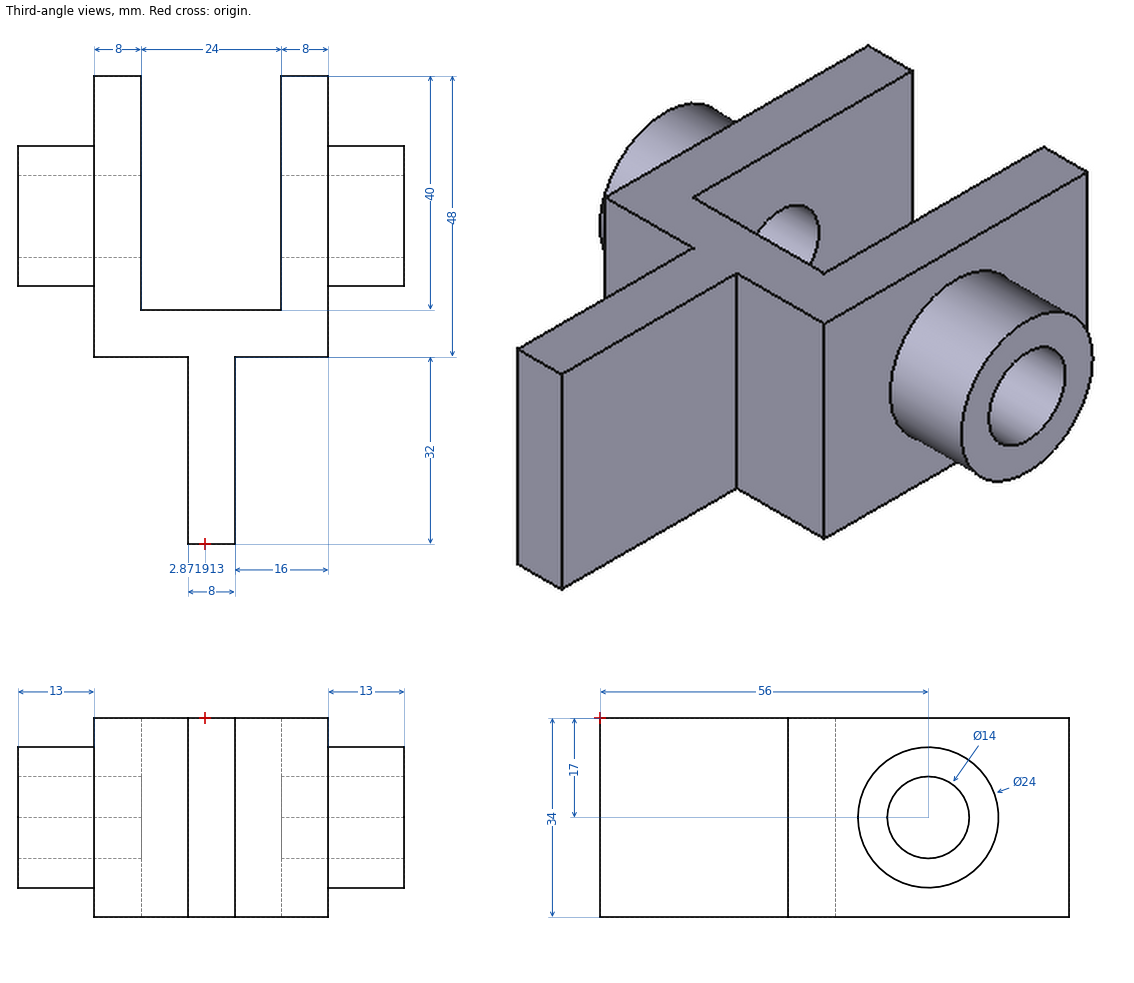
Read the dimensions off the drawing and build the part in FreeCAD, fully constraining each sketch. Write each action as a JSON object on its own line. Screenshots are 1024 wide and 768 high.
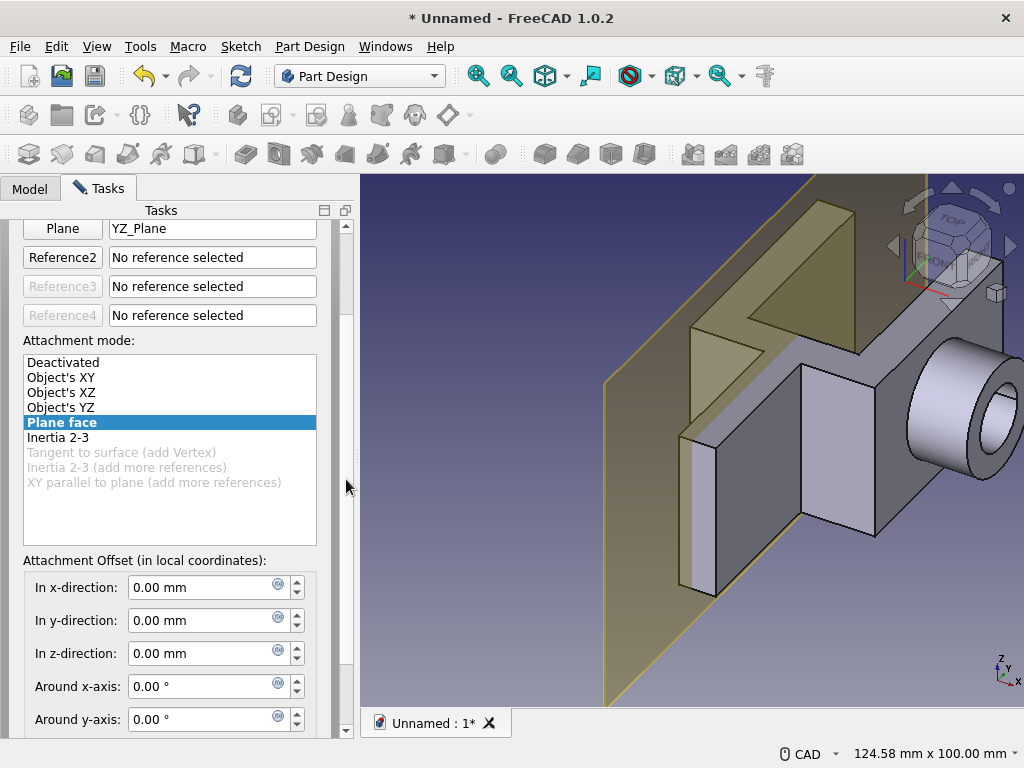
{"action": "triple_click", "coordinate": [210, 654]}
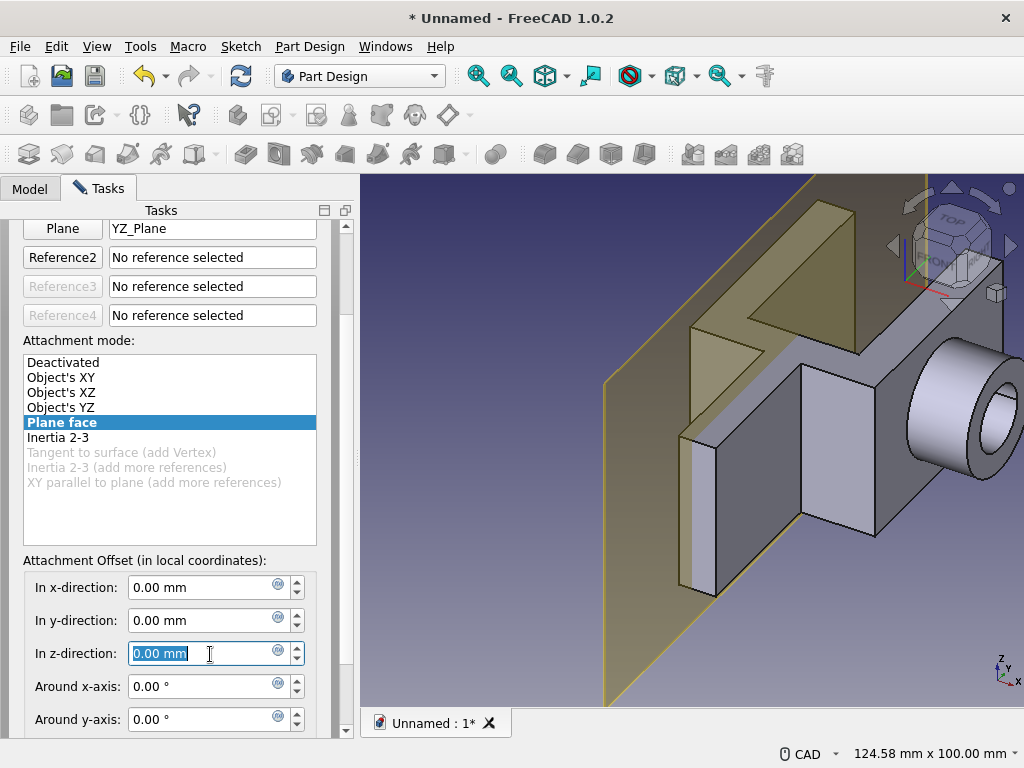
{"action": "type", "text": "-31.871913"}
{"action": "key", "text": "Tab"}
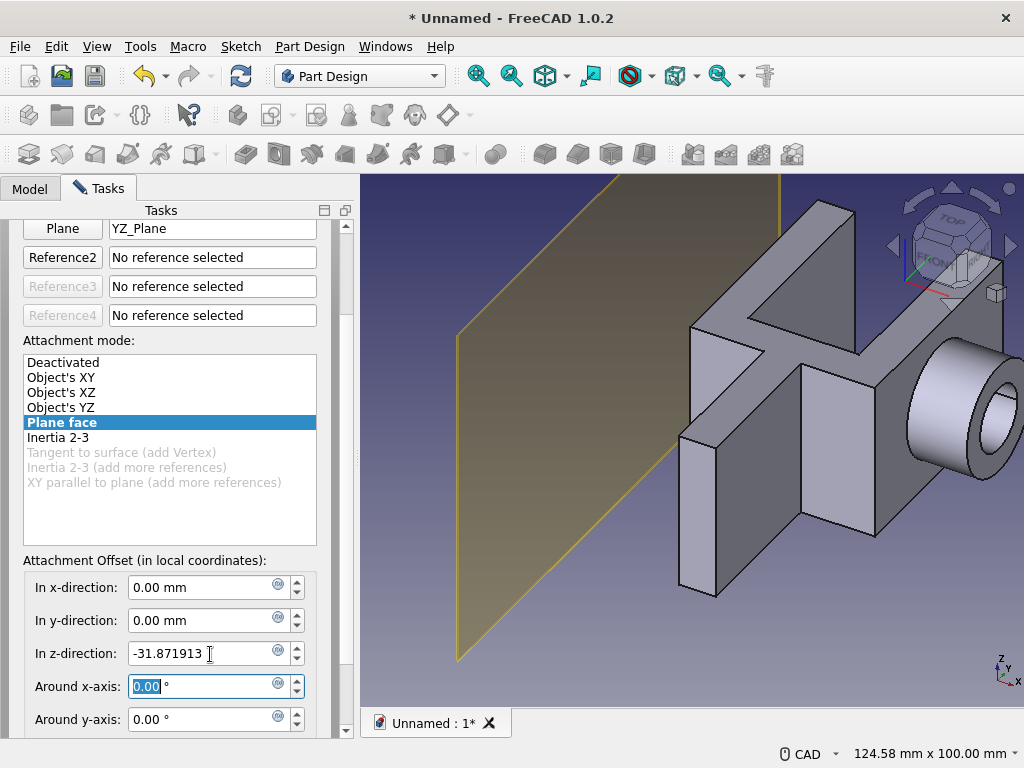
{"action": "scroll", "coordinate": [346, 479], "scroll_direction": "up", "scroll_amount": 3}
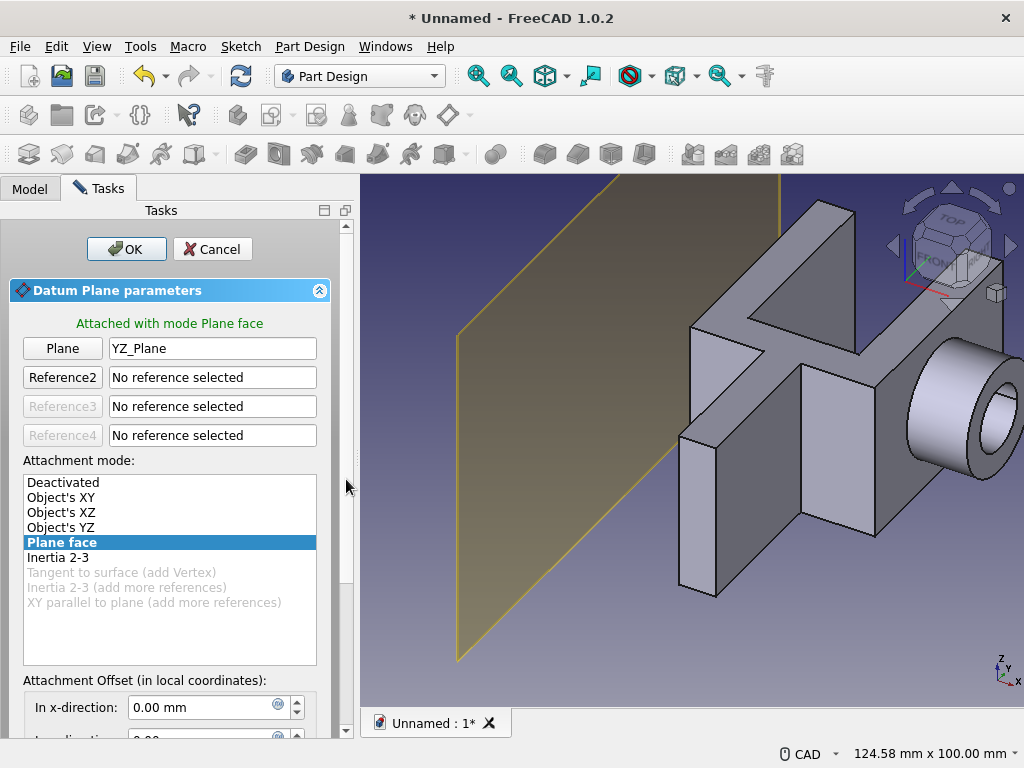
{"action": "left_click", "coordinate": [127, 249]}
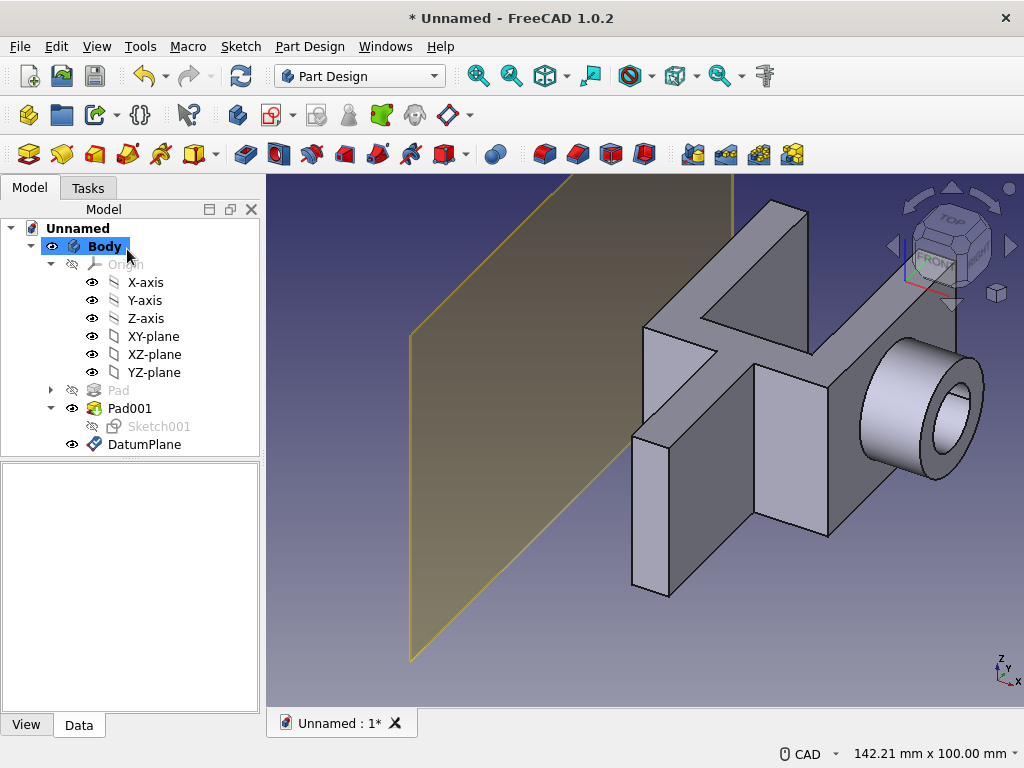
{"action": "left_click", "coordinate": [117, 444]}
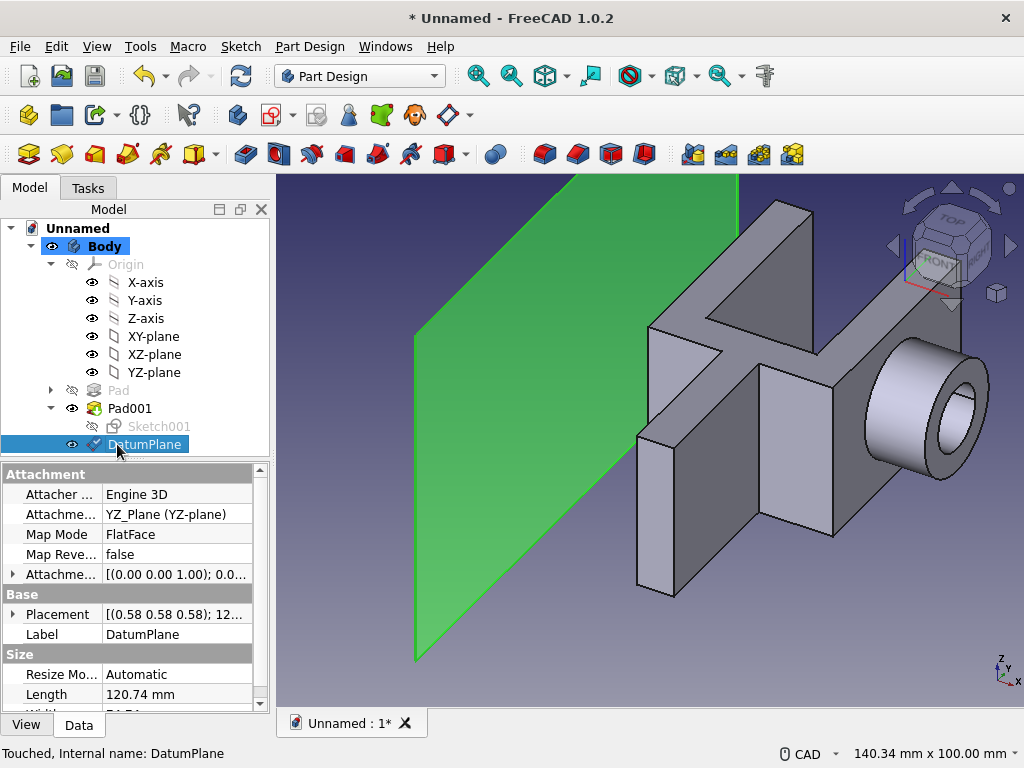
{"action": "left_click", "coordinate": [270, 116]}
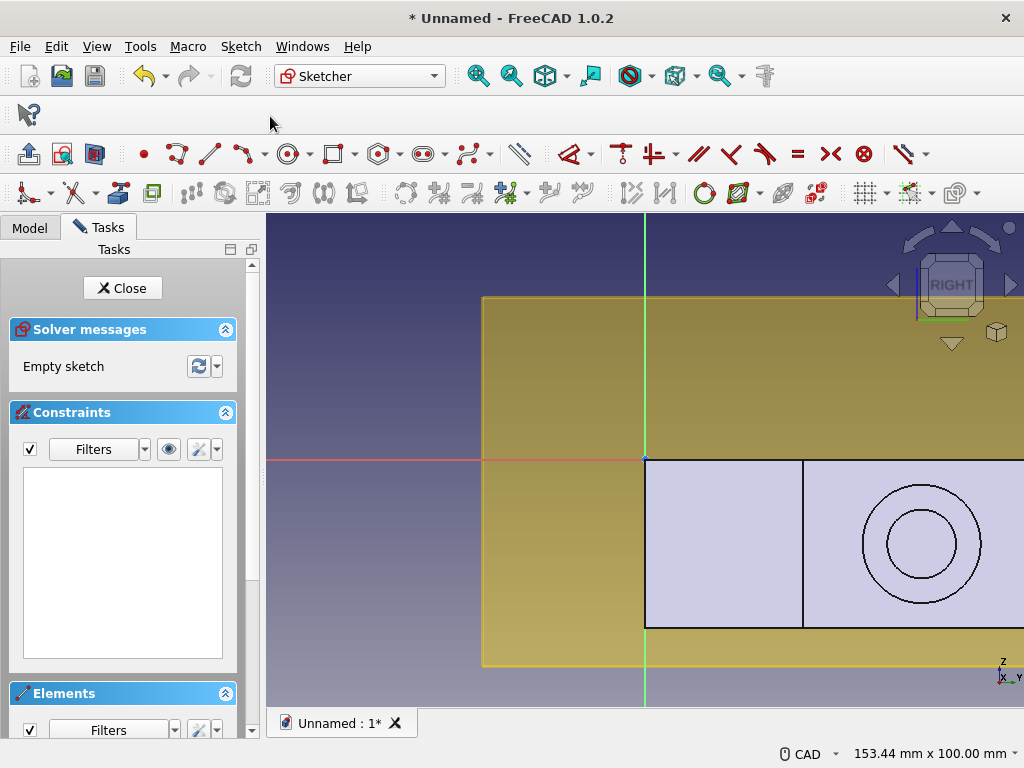
{"action": "key", "text": "q s"}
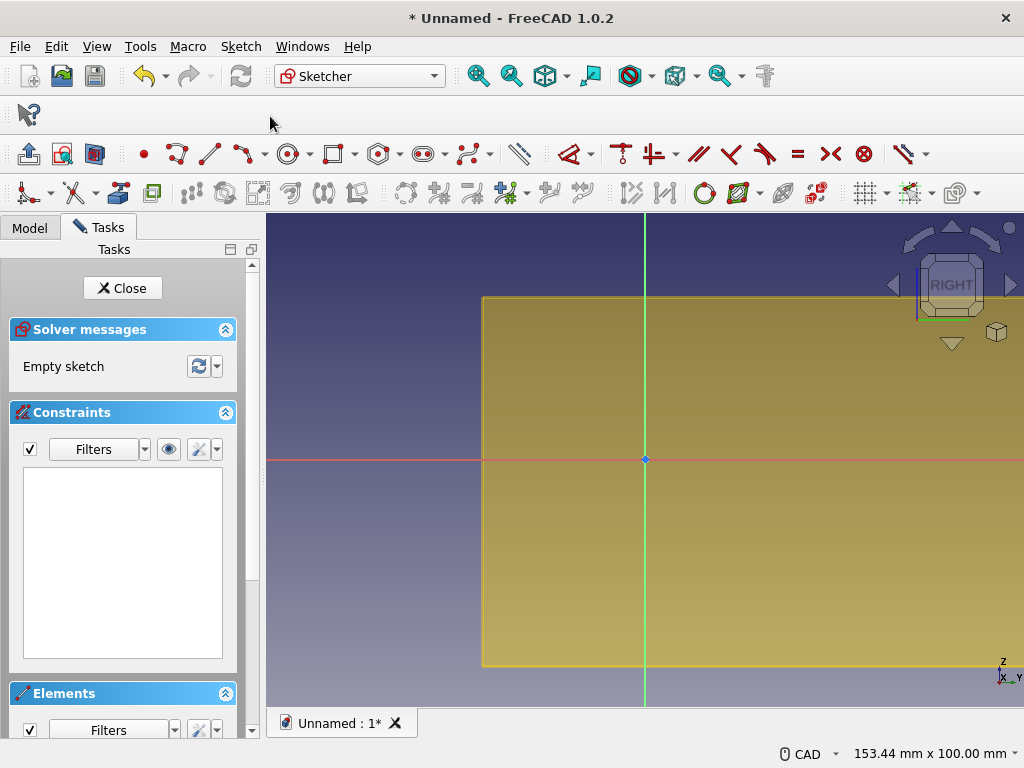
{"action": "scroll", "coordinate": [576, 460], "scroll_direction": "down", "scroll_amount": 5}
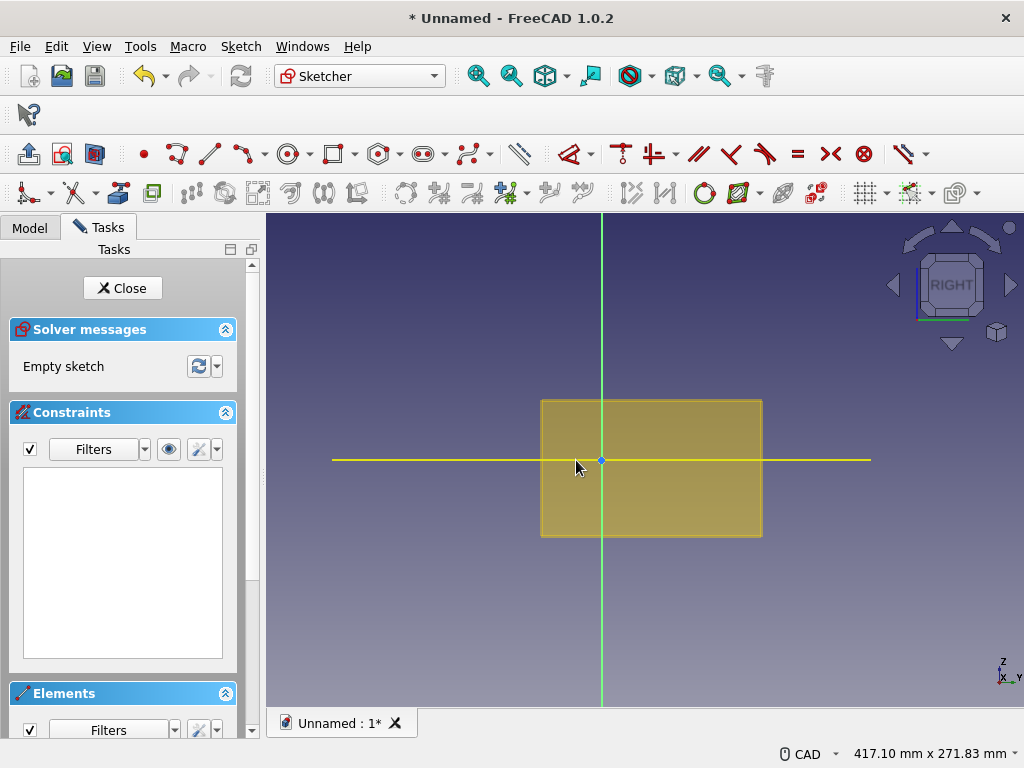
{"action": "scroll", "coordinate": [723, 496], "scroll_direction": "up", "scroll_amount": 10}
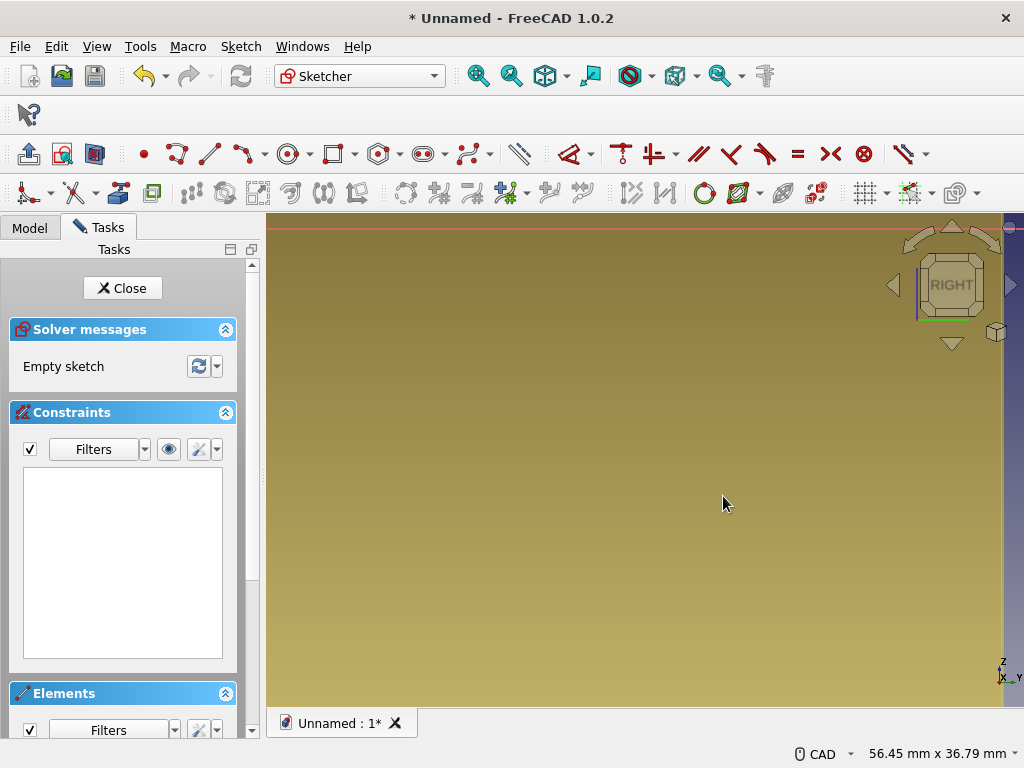
{"action": "key", "text": "g c"}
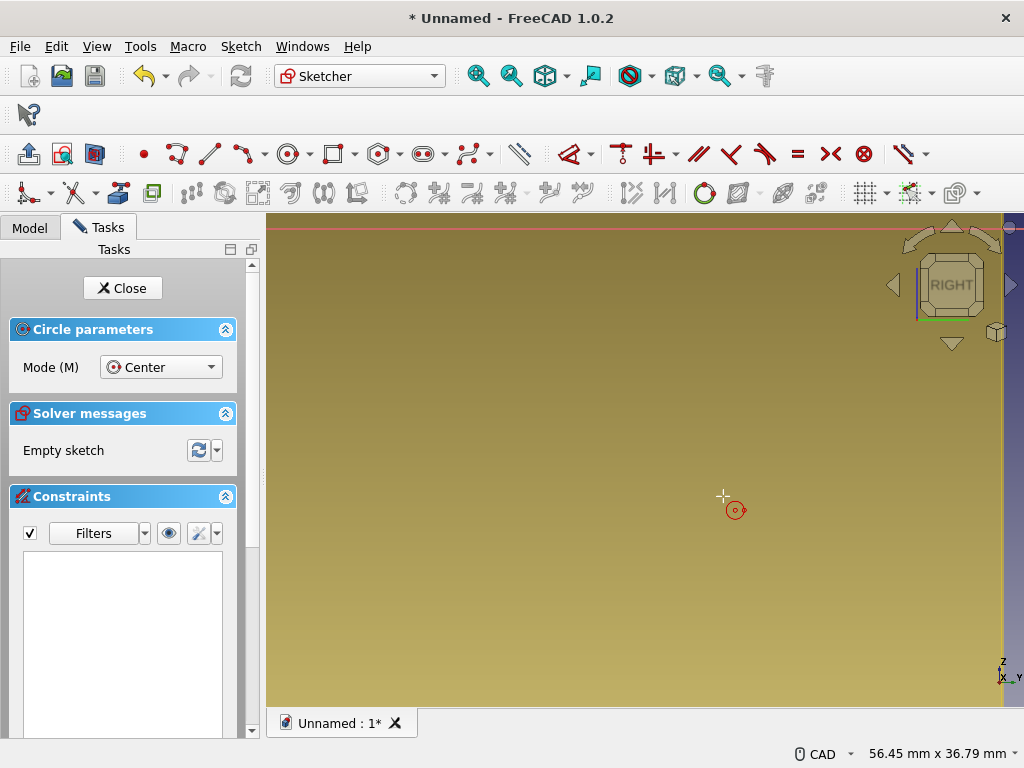
{"action": "left_click", "coordinate": [574, 457]}
{"action": "mouse_move", "coordinate": [688, 343]}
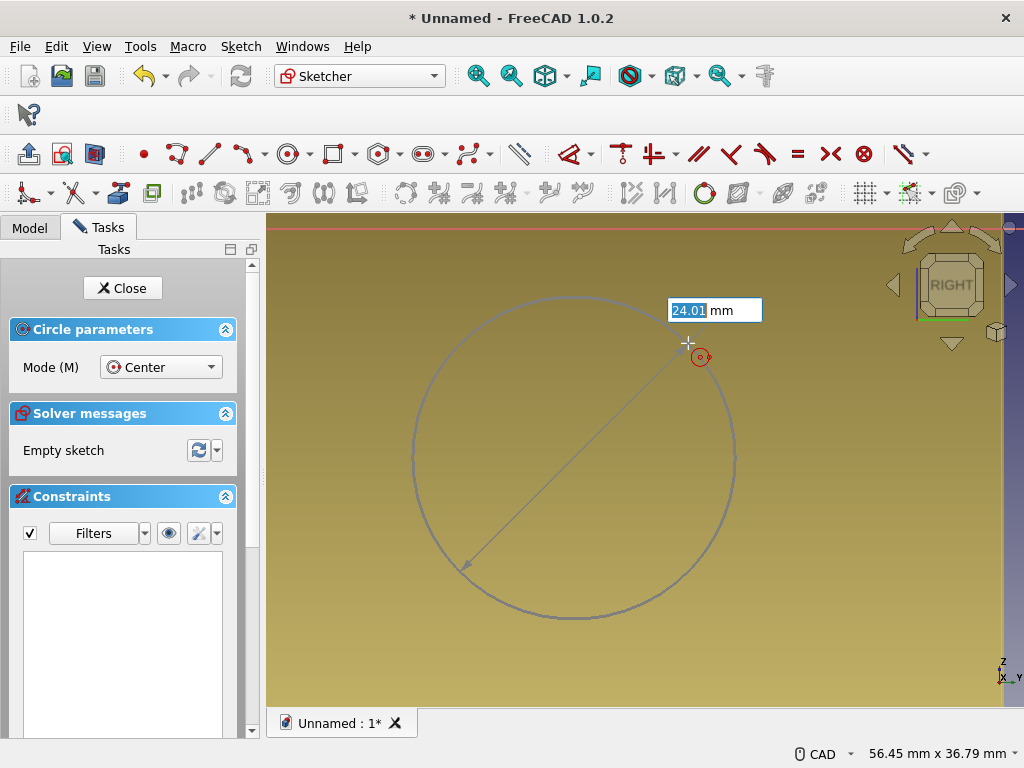
{"action": "type", "text": "24"}
{"action": "key", "text": "Return"}